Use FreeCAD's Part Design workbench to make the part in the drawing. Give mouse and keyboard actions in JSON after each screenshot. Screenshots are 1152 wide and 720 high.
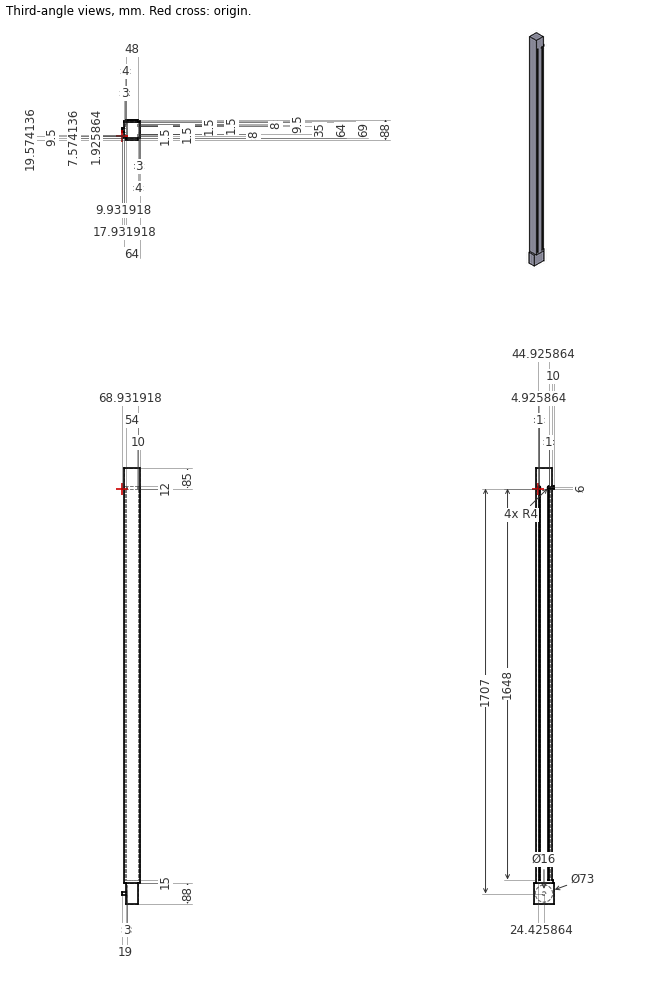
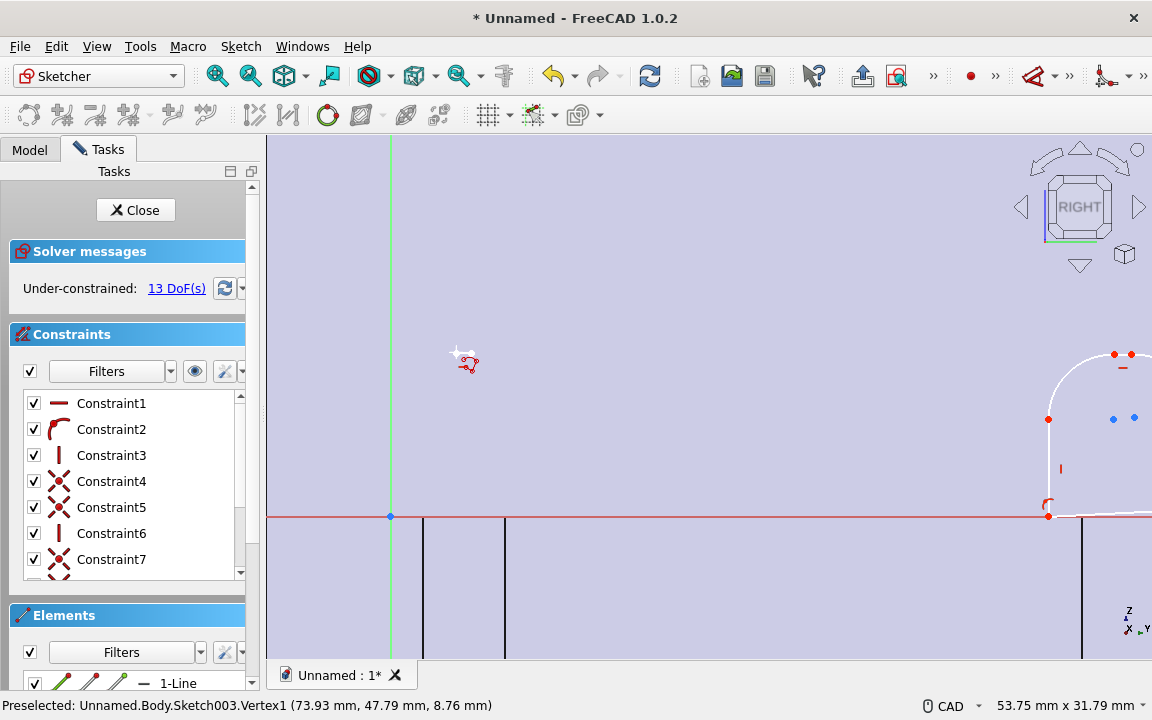
{"action": "scroll", "coordinate": [390, 418], "scroll_direction": "up", "scroll_amount": 13}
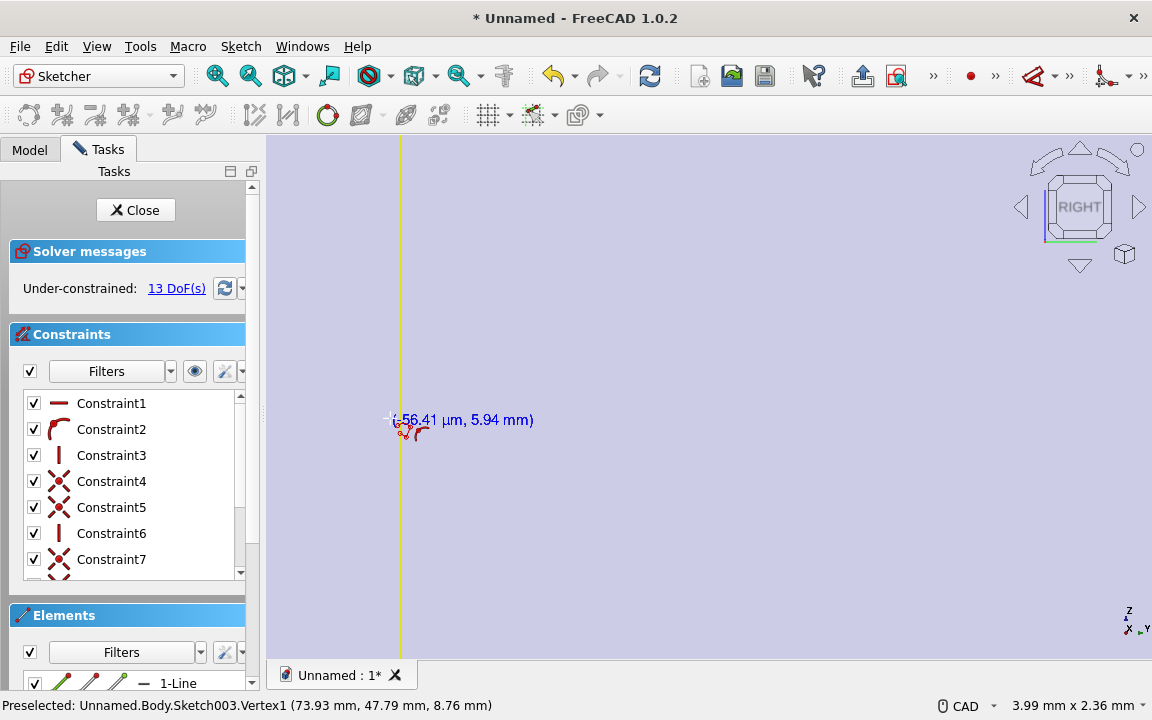
{"action": "left_click", "coordinate": [384, 412]}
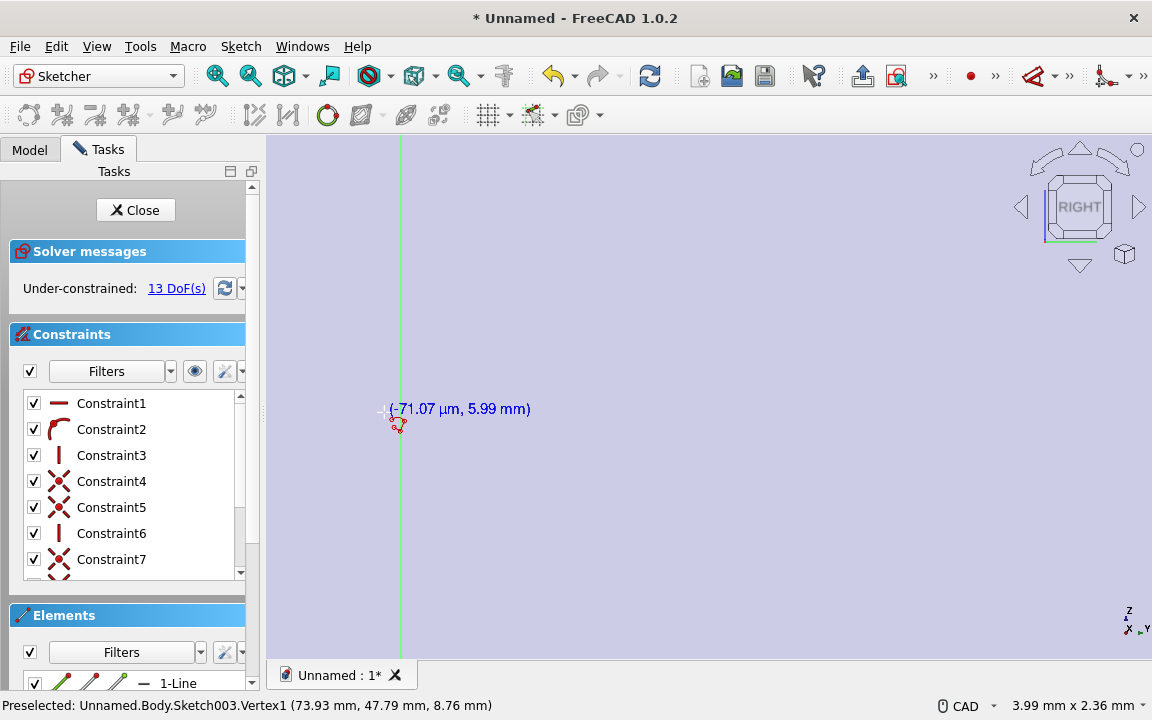
{"action": "scroll", "coordinate": [369, 385], "scroll_direction": "down", "scroll_amount": 15}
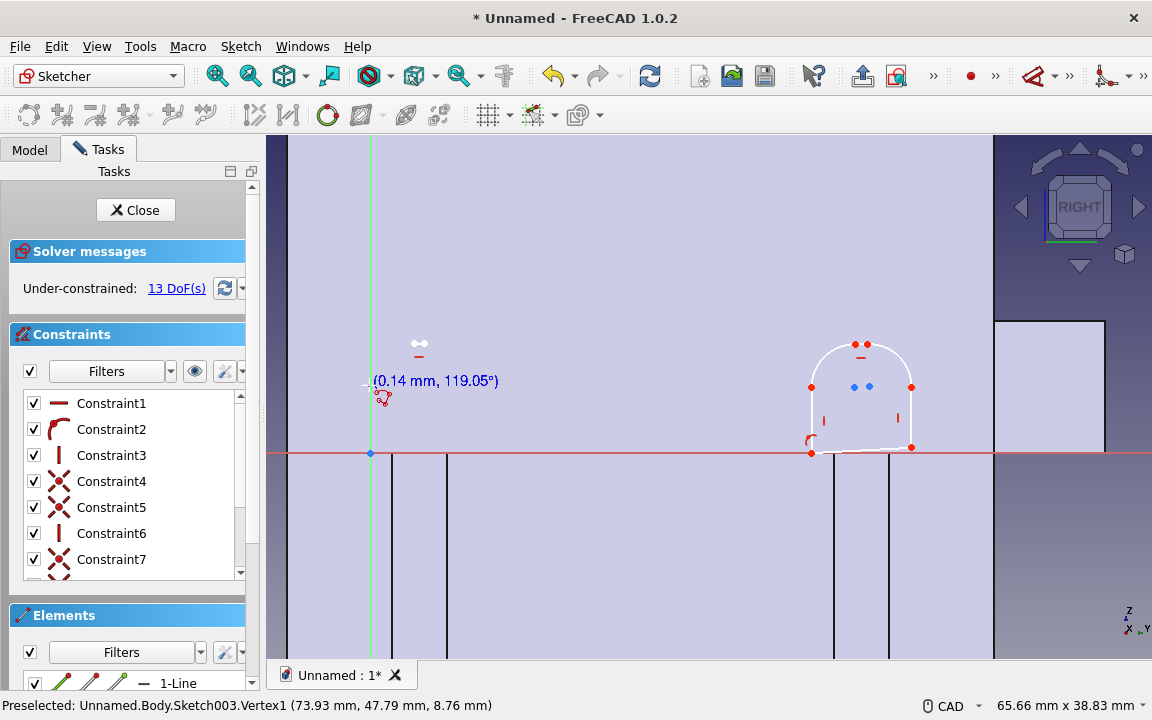
{"action": "scroll", "coordinate": [370, 453], "scroll_direction": "up", "scroll_amount": 15}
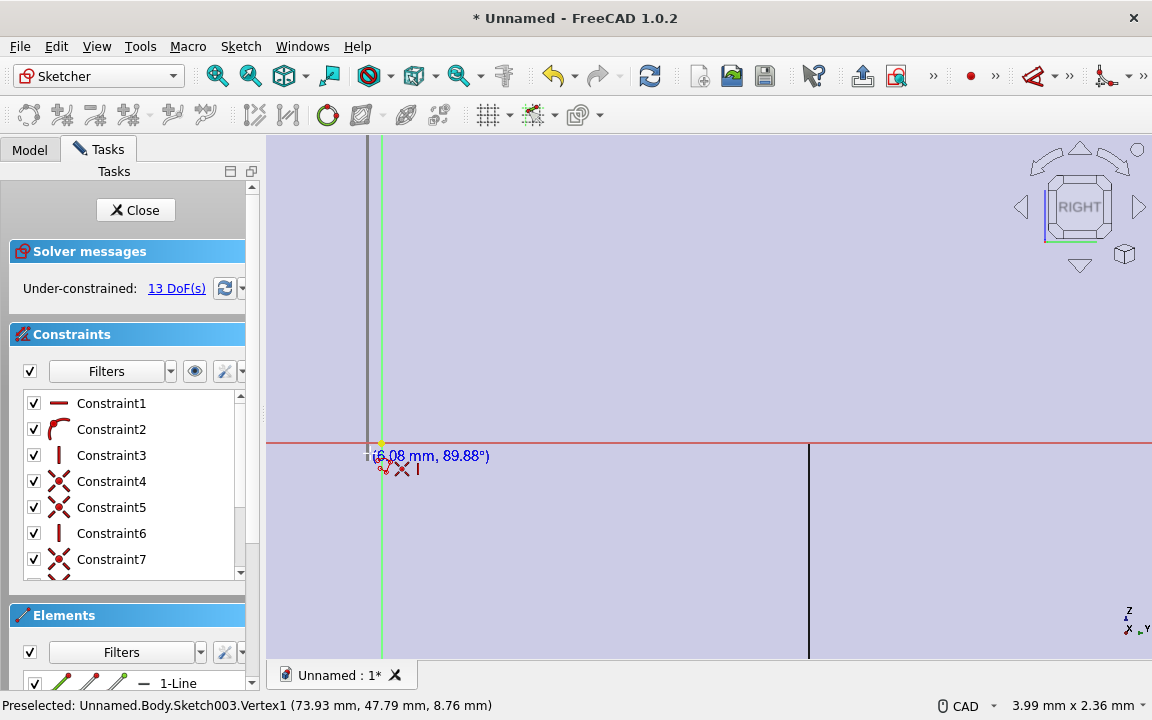
{"action": "left_click", "coordinate": [365, 443]}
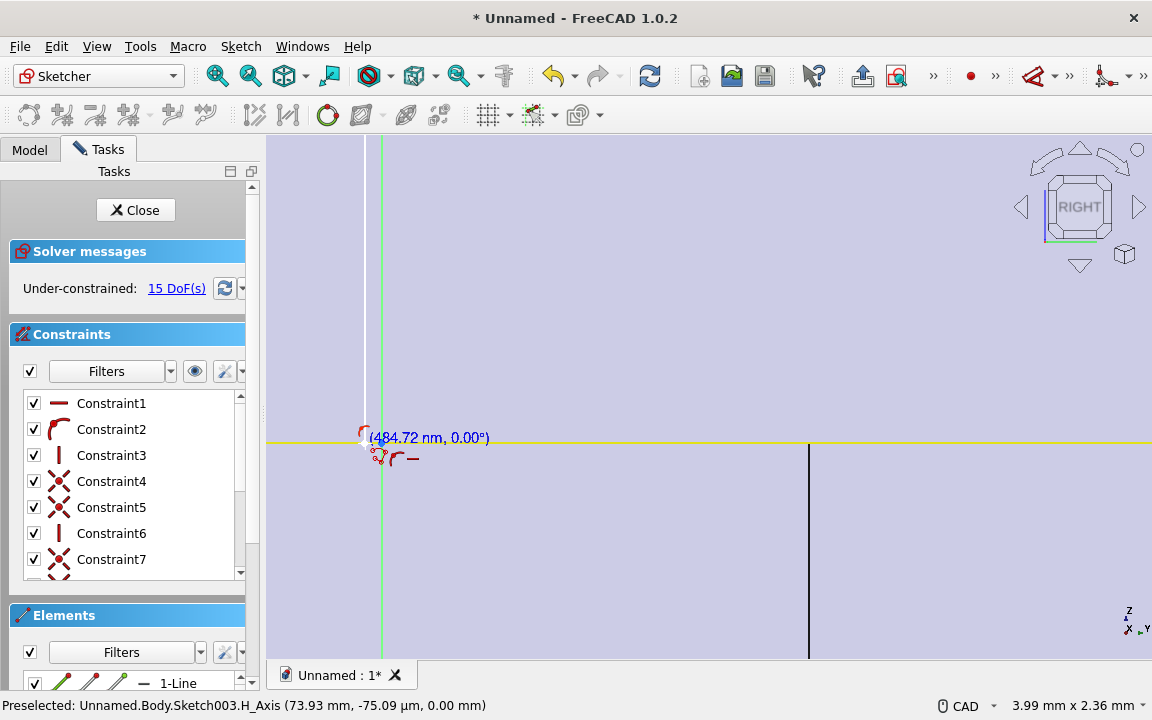
{"action": "scroll", "coordinate": [370, 453], "scroll_direction": "down", "scroll_amount": 15}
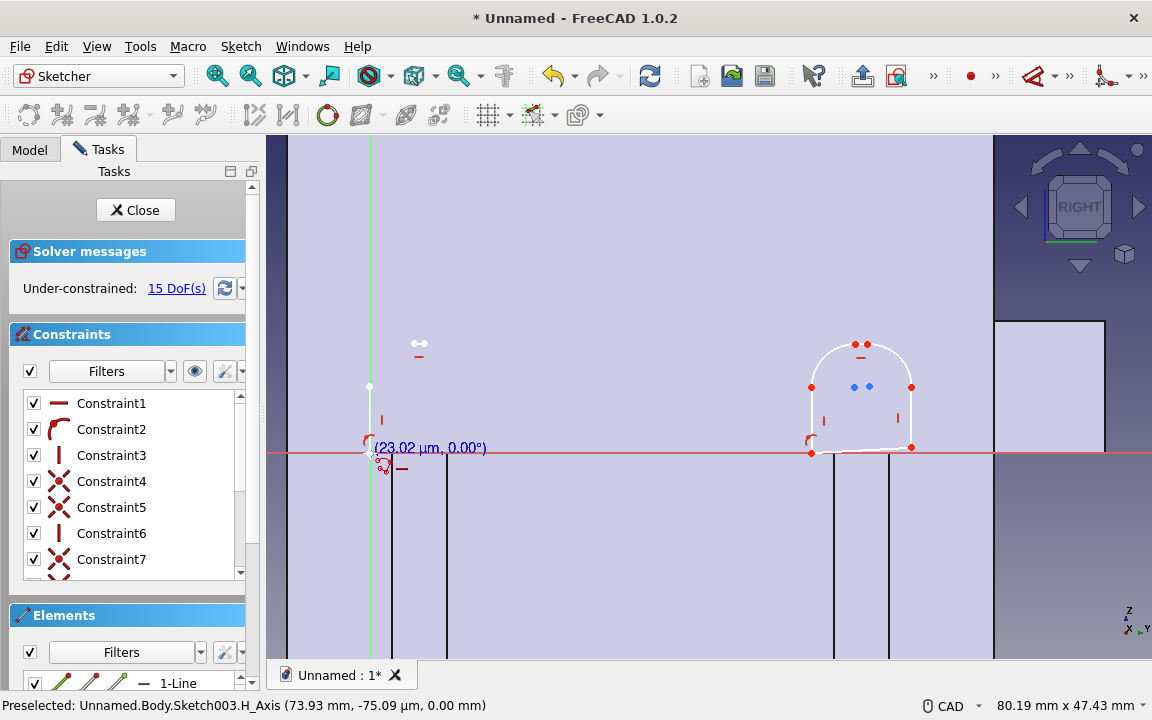
{"action": "left_click", "coordinate": [469, 444]}
{"action": "left_click", "coordinate": [469, 387]}
{"action": "right_click", "coordinate": [469, 387]}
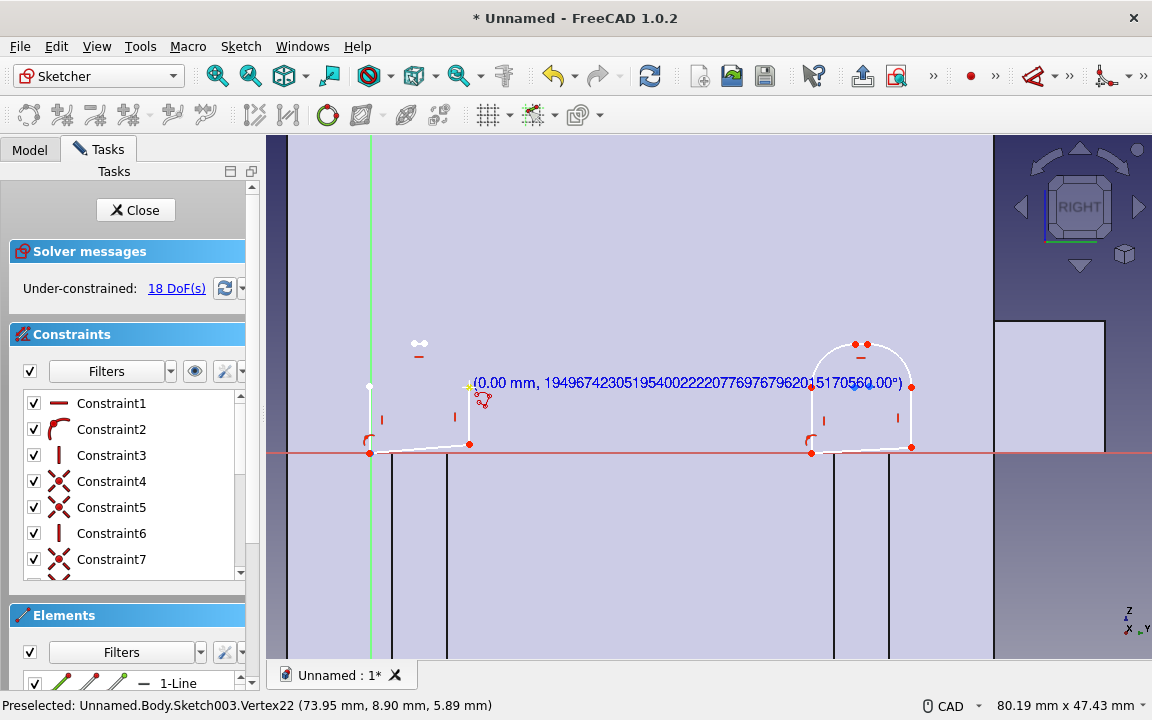
{"action": "key", "text": "g 3 a"}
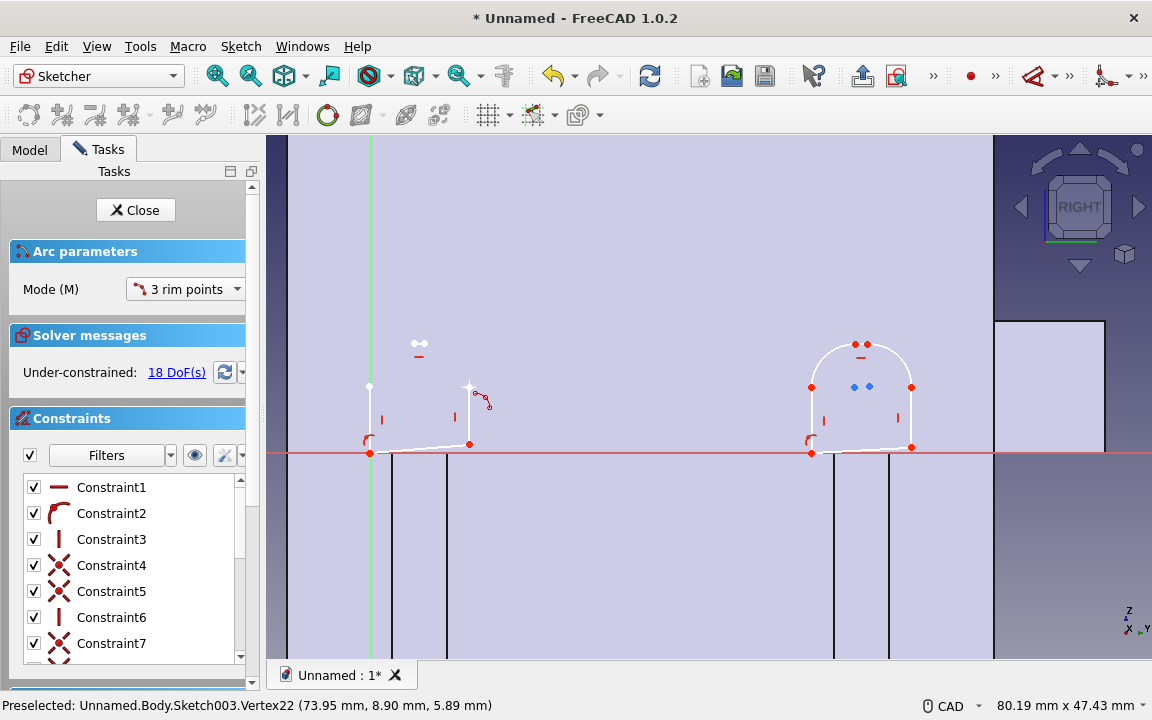
{"action": "scroll", "coordinate": [414, 343], "scroll_direction": "up", "scroll_amount": 6}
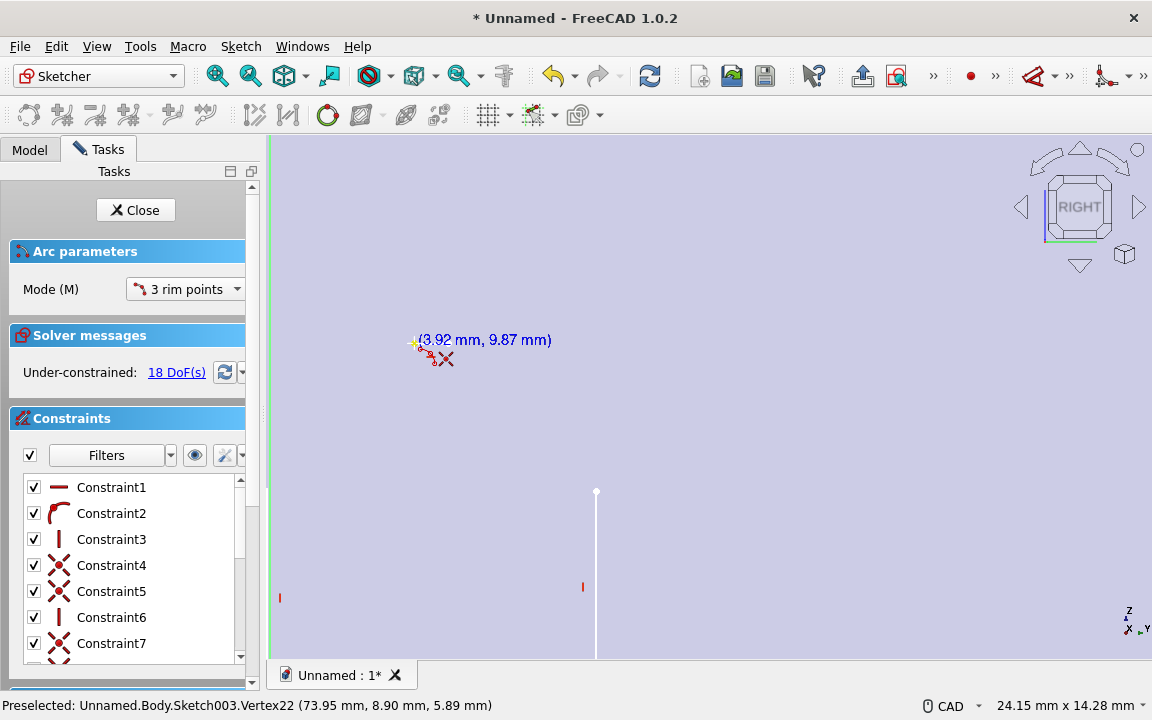
{"action": "left_click", "coordinate": [415, 344]}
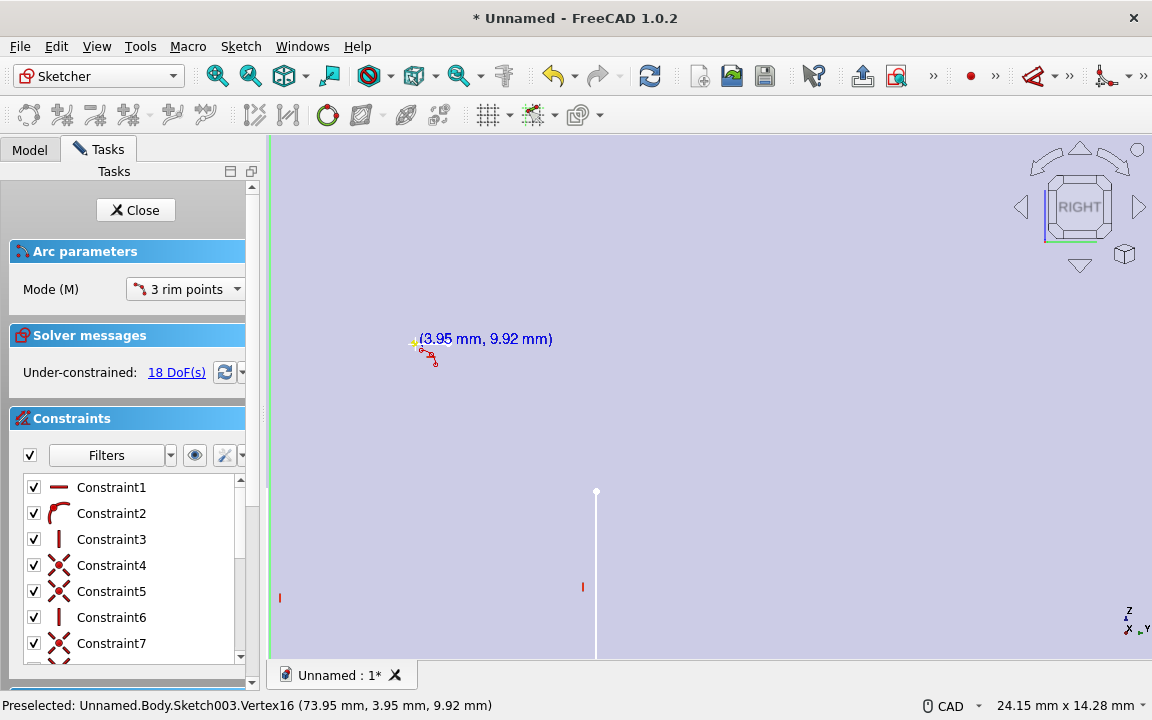
{"action": "scroll", "coordinate": [469, 355], "scroll_direction": "down", "scroll_amount": 7}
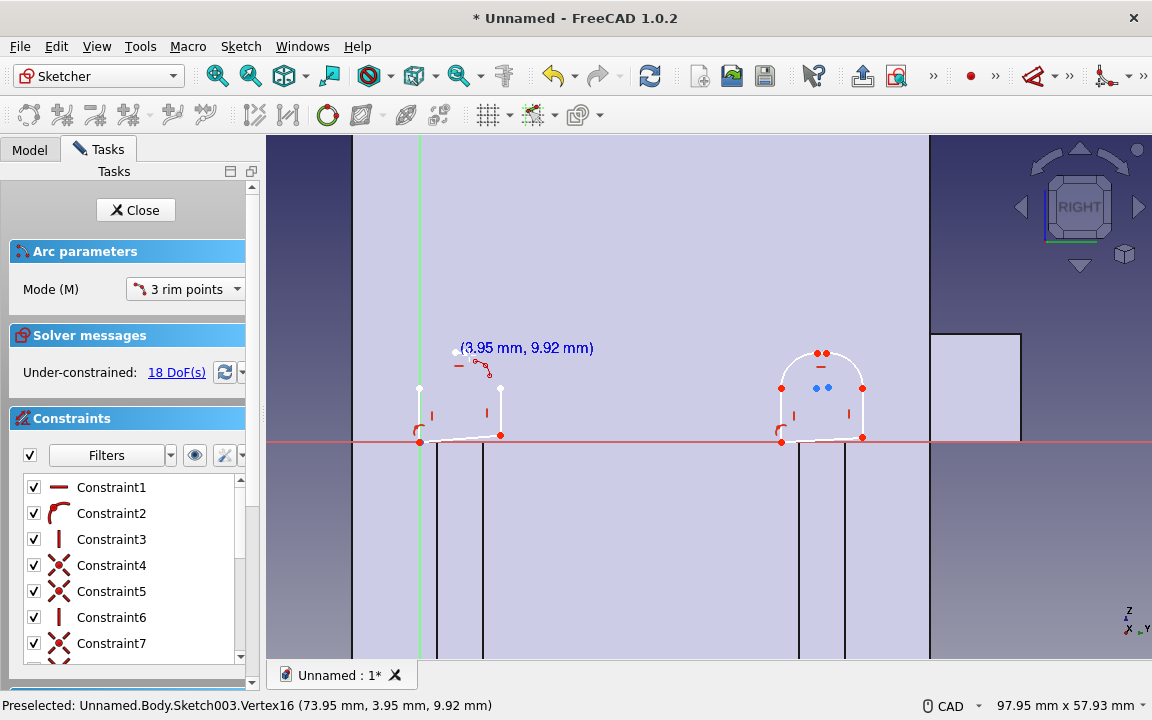
{"action": "scroll", "coordinate": [419, 388], "scroll_direction": "up", "scroll_amount": 16}